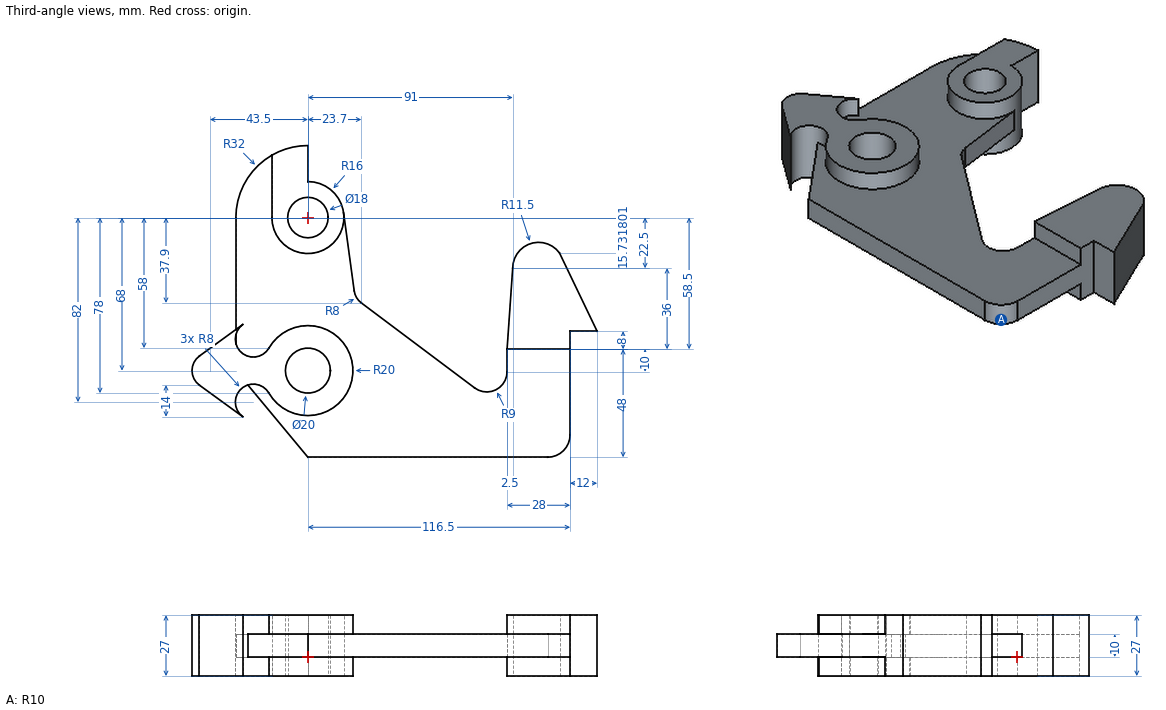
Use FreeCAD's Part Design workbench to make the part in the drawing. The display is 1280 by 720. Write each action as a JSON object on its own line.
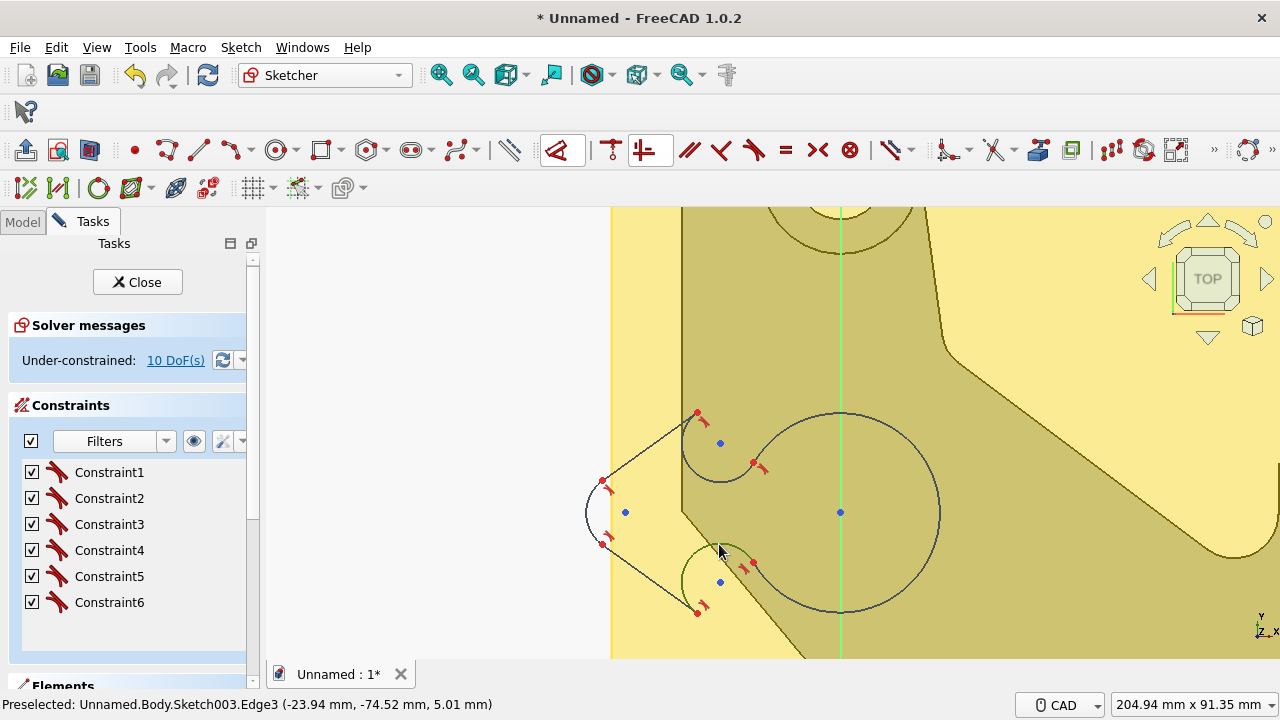
{"action": "left_click", "coordinate": [682, 448]}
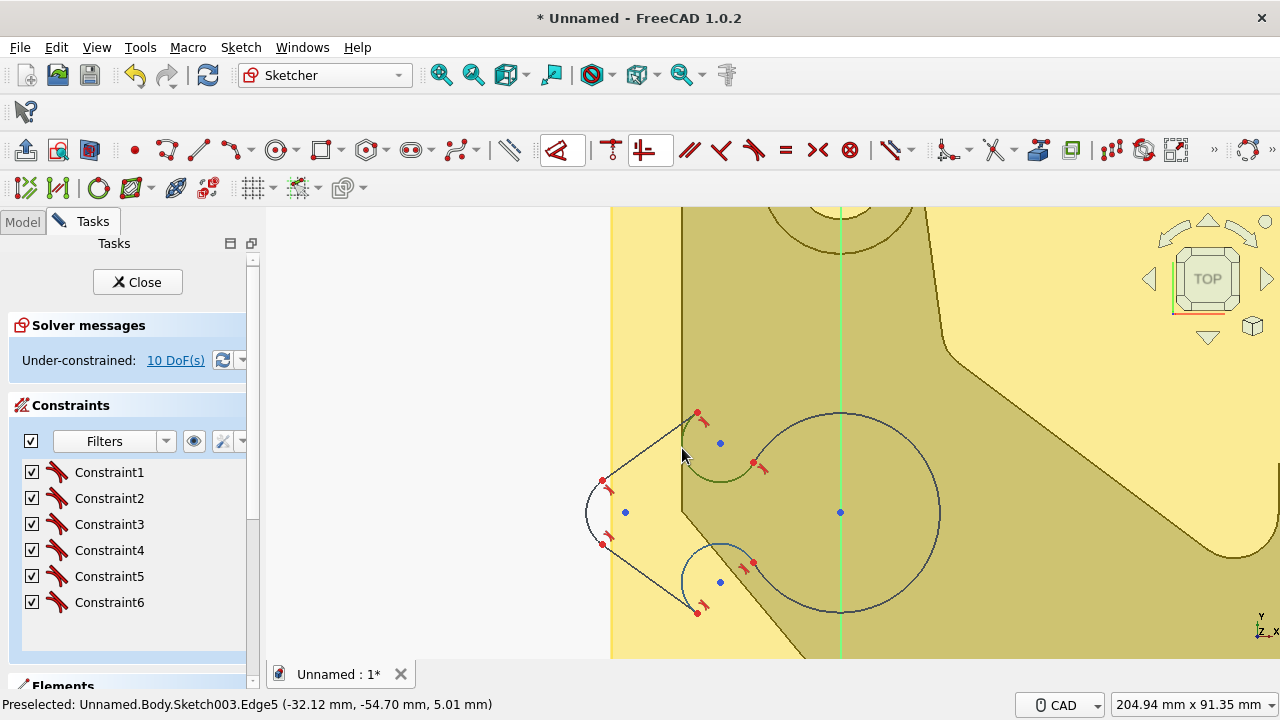
{"action": "left_click", "coordinate": [589, 498]}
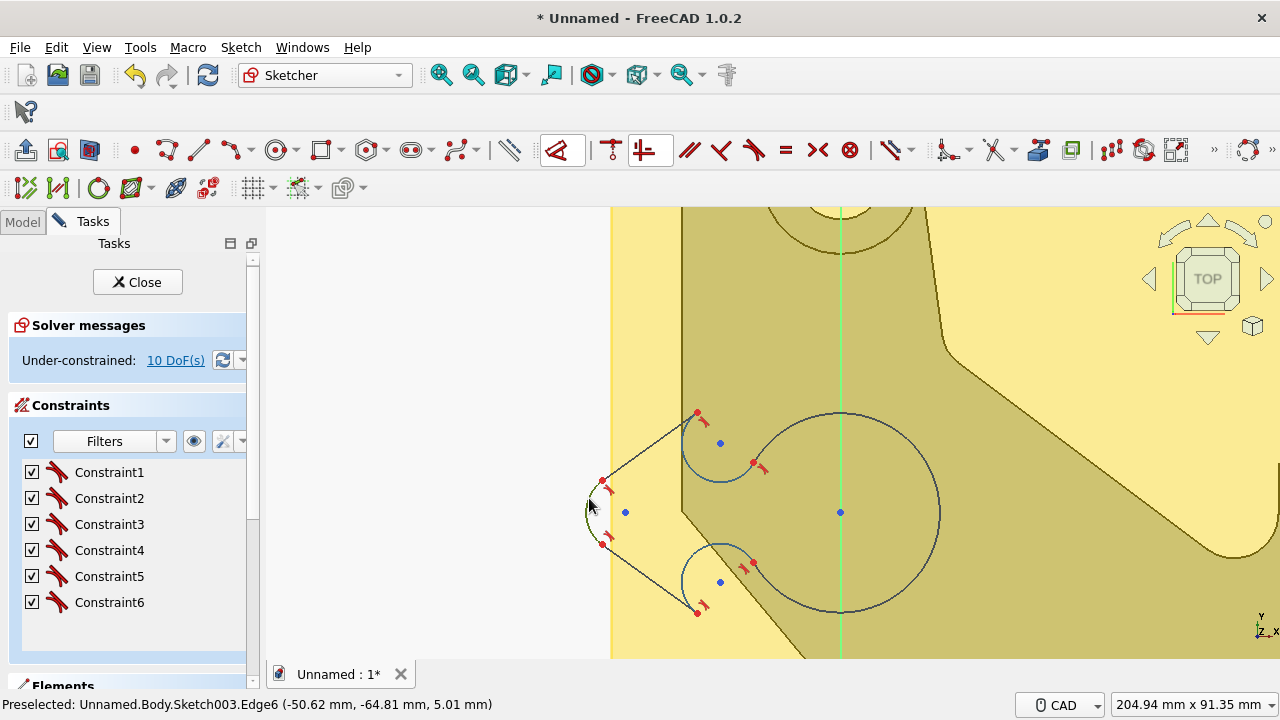
{"action": "left_click", "coordinate": [786, 150]}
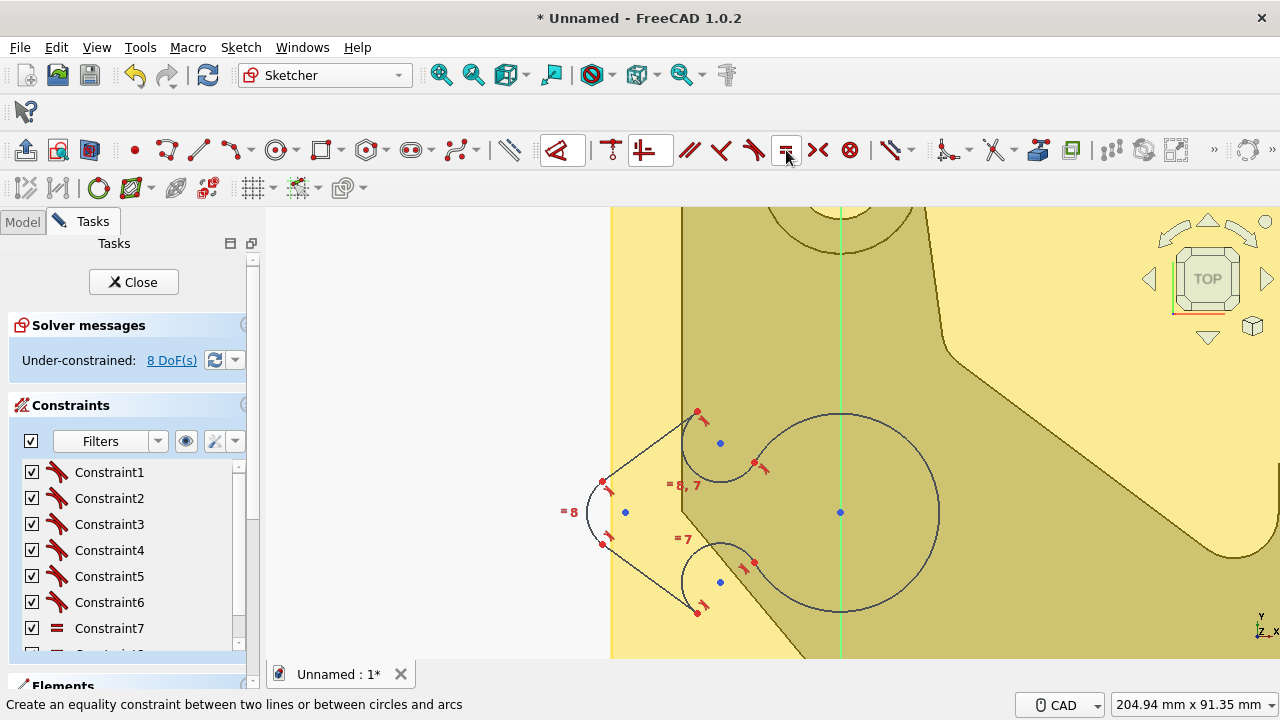
{"action": "left_click", "coordinate": [840, 513]}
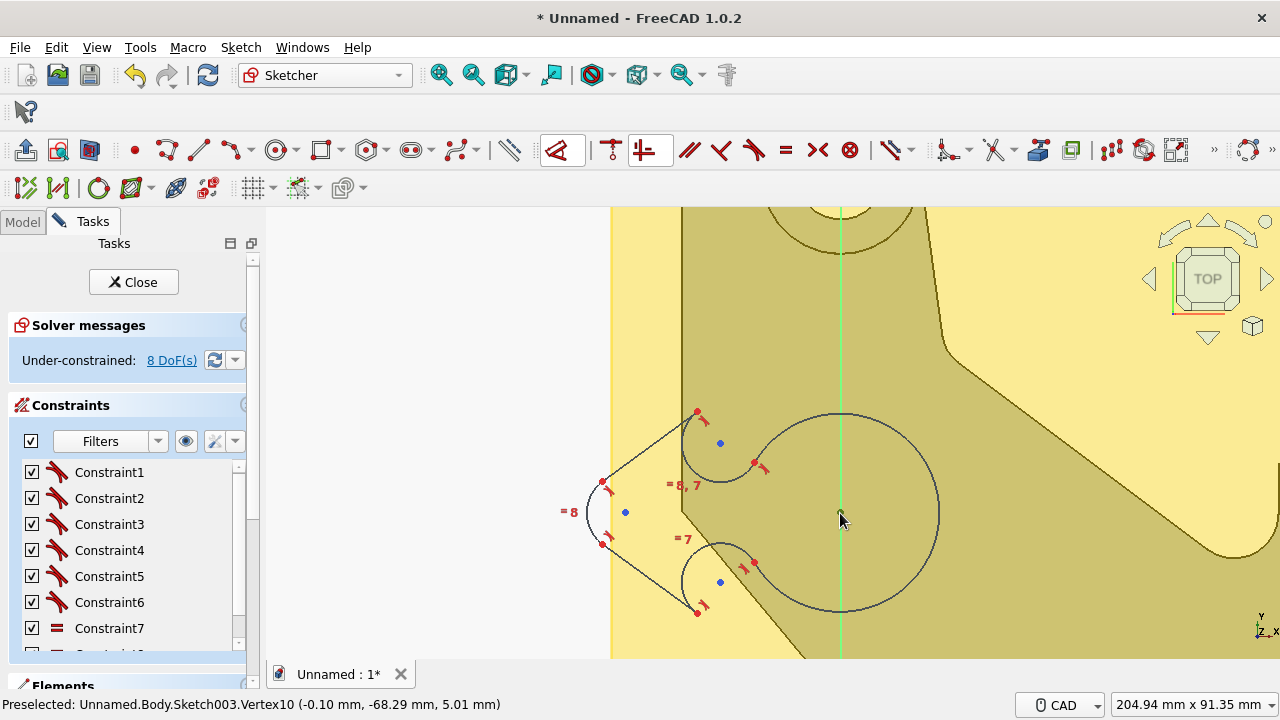
{"action": "left_click", "coordinate": [841, 574]}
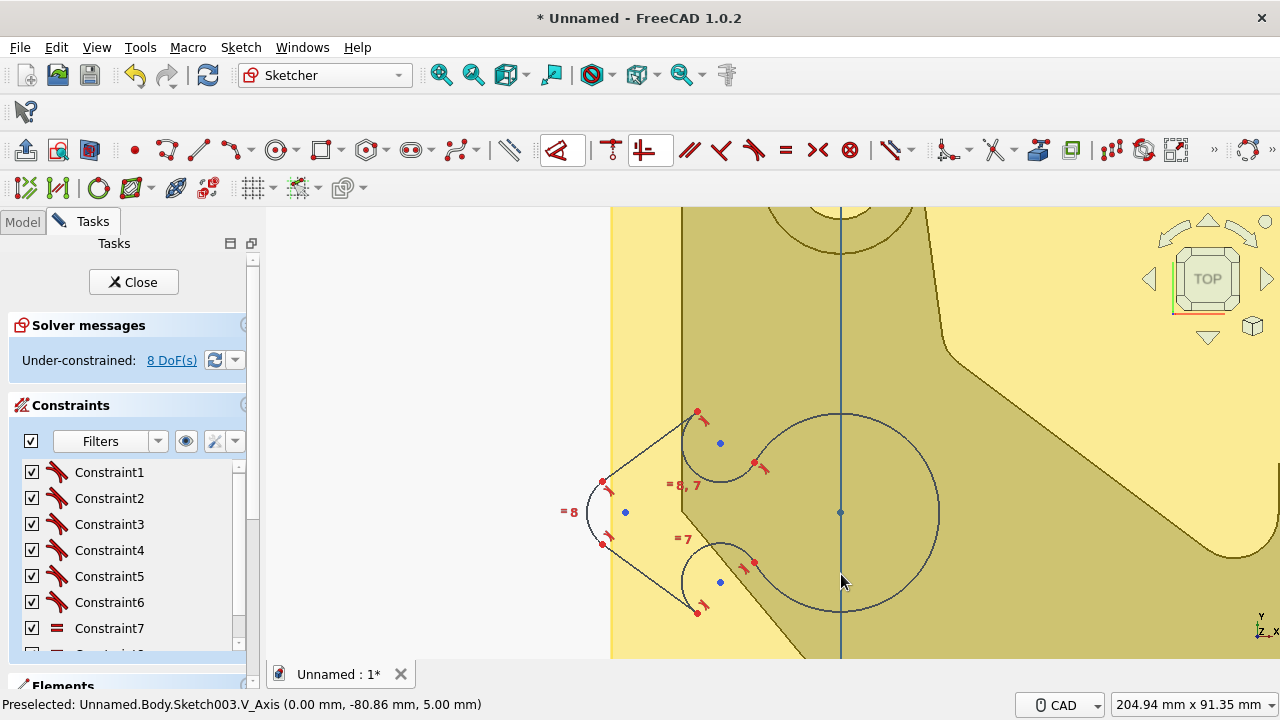
{"action": "left_click", "coordinate": [612, 150]}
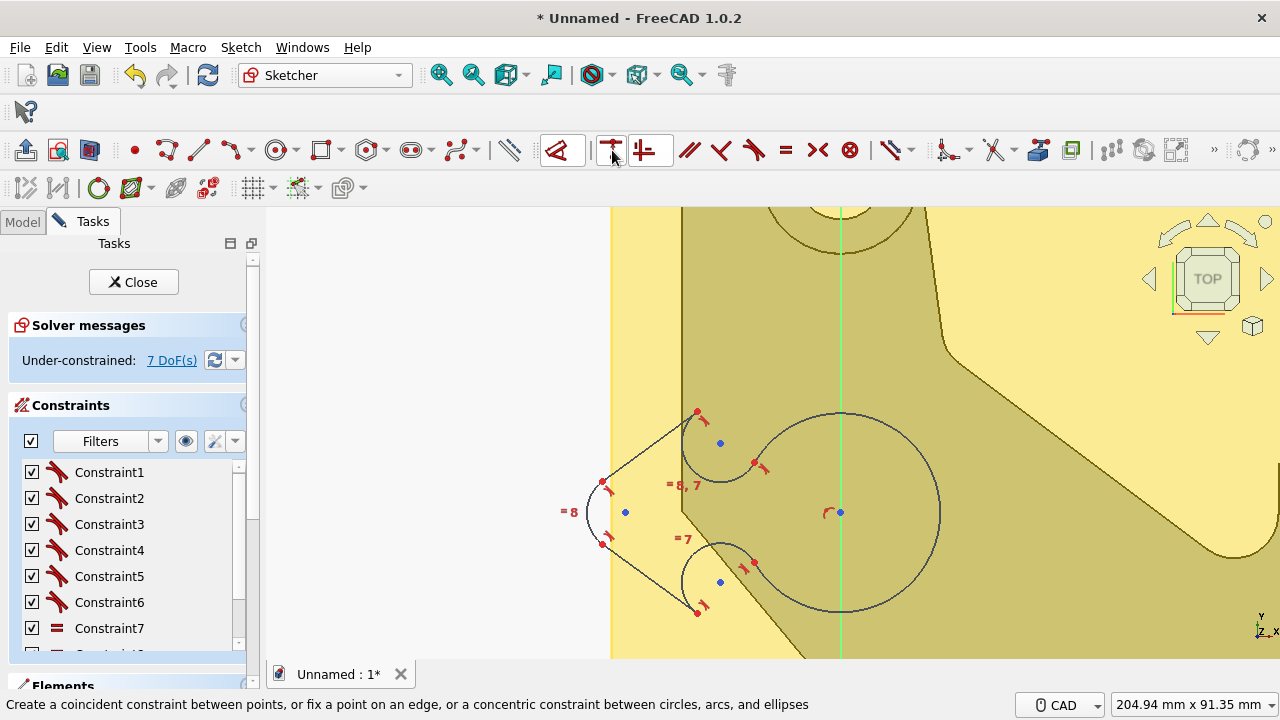
{"action": "left_click", "coordinate": [720, 543]}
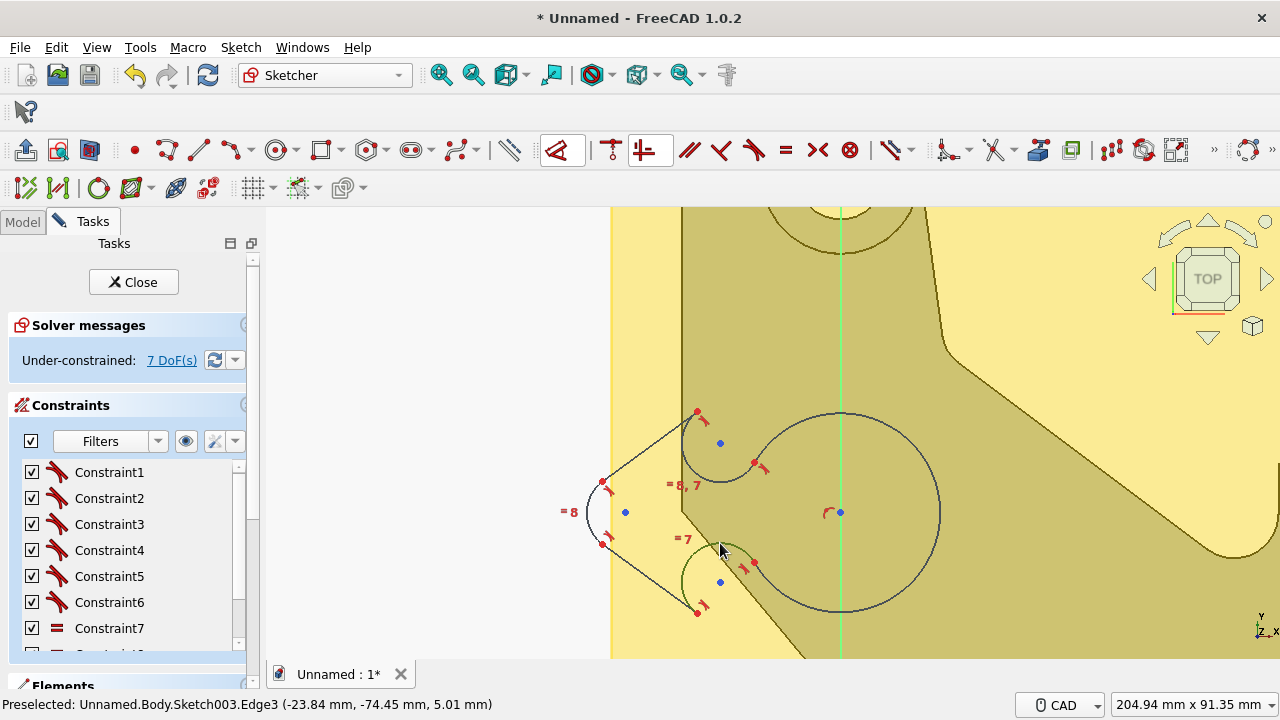
{"action": "left_click", "coordinate": [580, 150]}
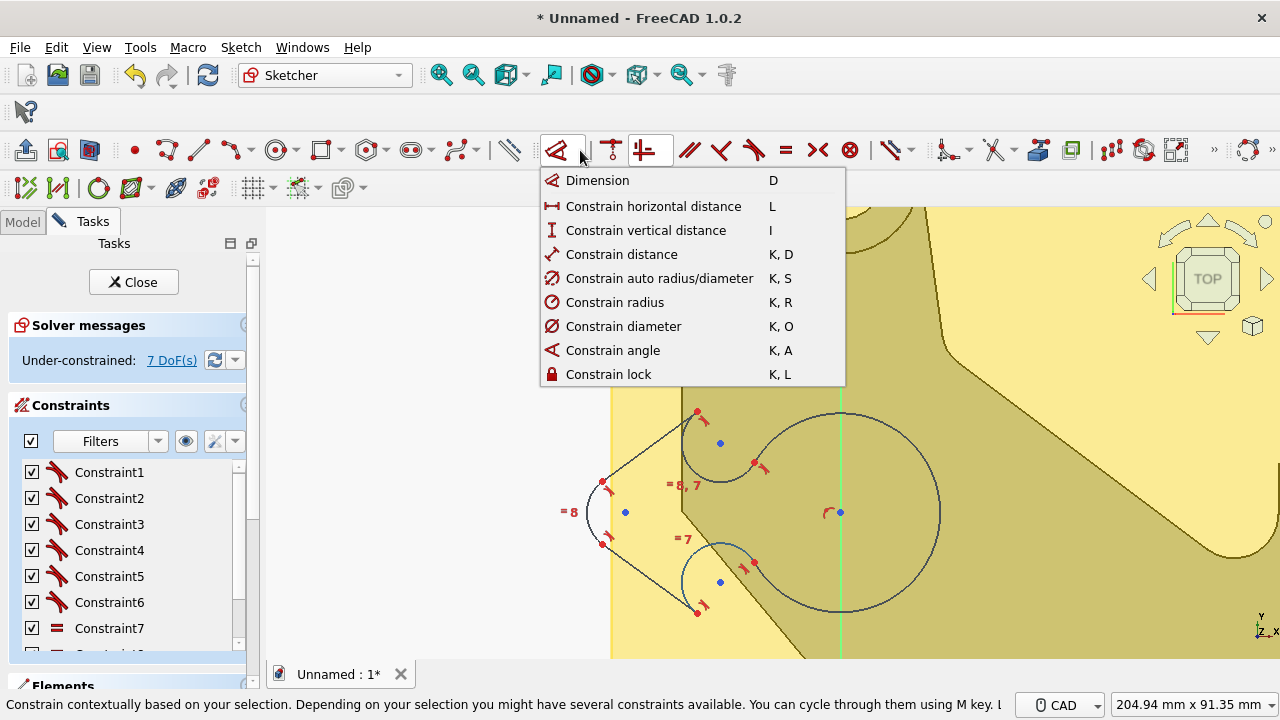
{"action": "left_click", "coordinate": [693, 302]}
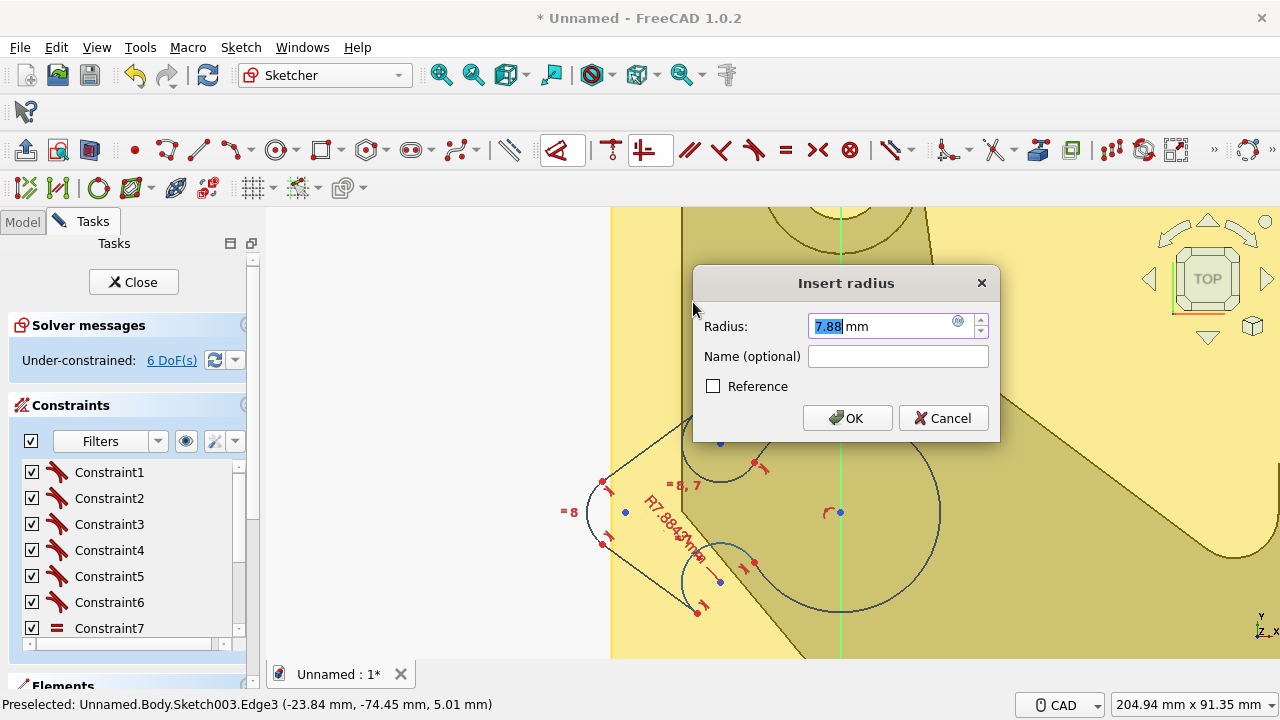
{"action": "type", "text": "8"}
{"action": "key", "text": "Return"}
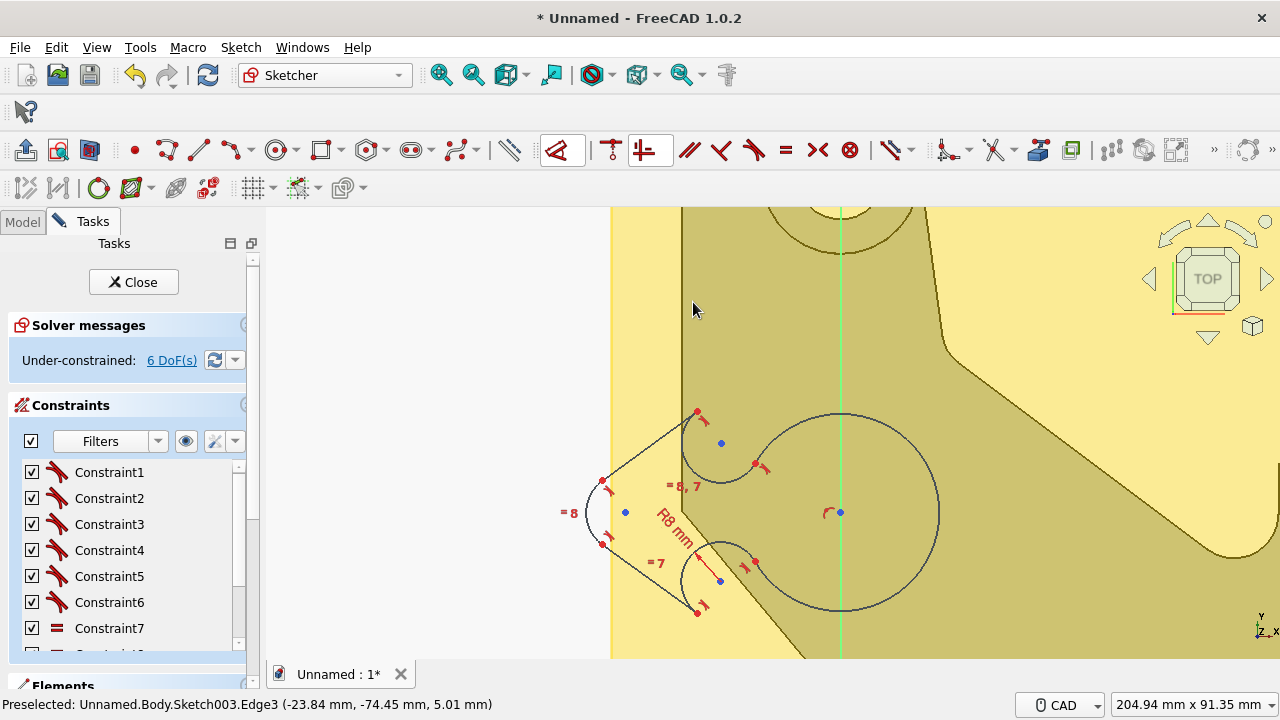
{"action": "left_click", "coordinate": [890, 598]}